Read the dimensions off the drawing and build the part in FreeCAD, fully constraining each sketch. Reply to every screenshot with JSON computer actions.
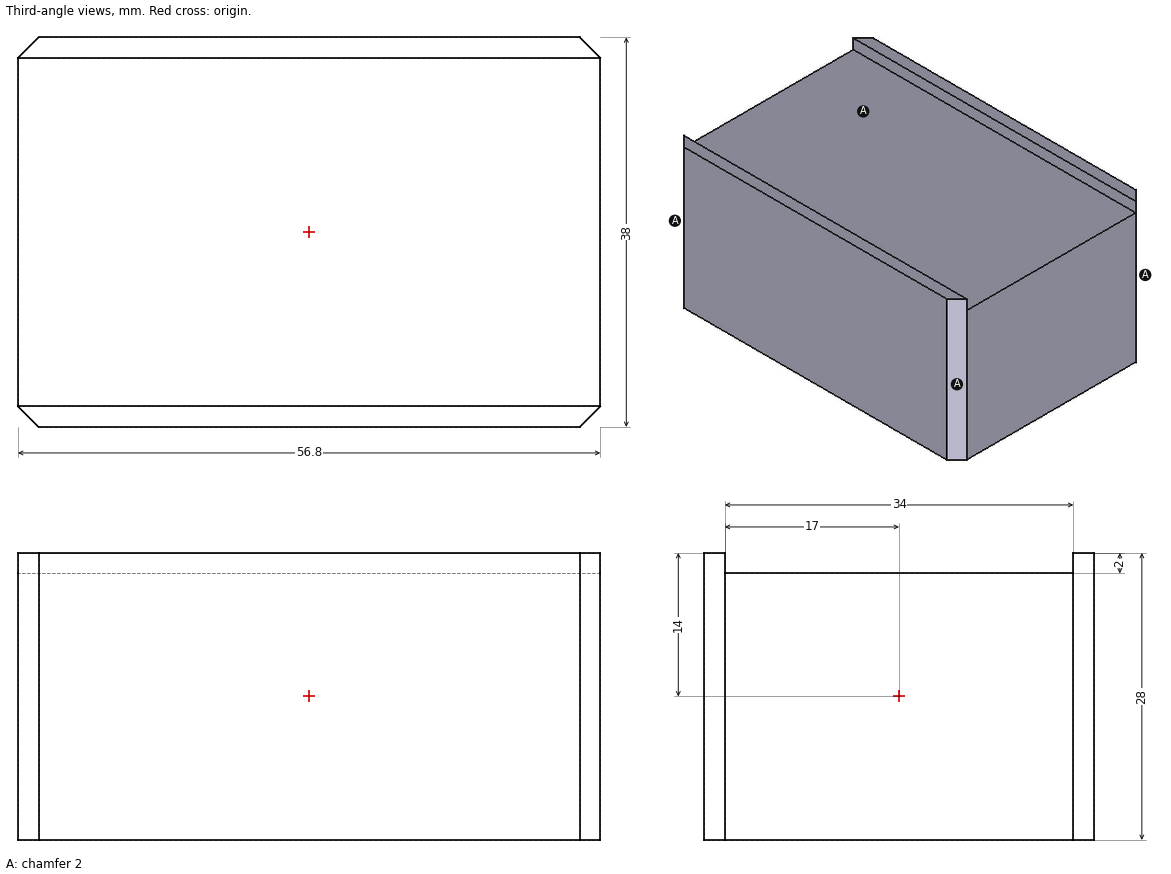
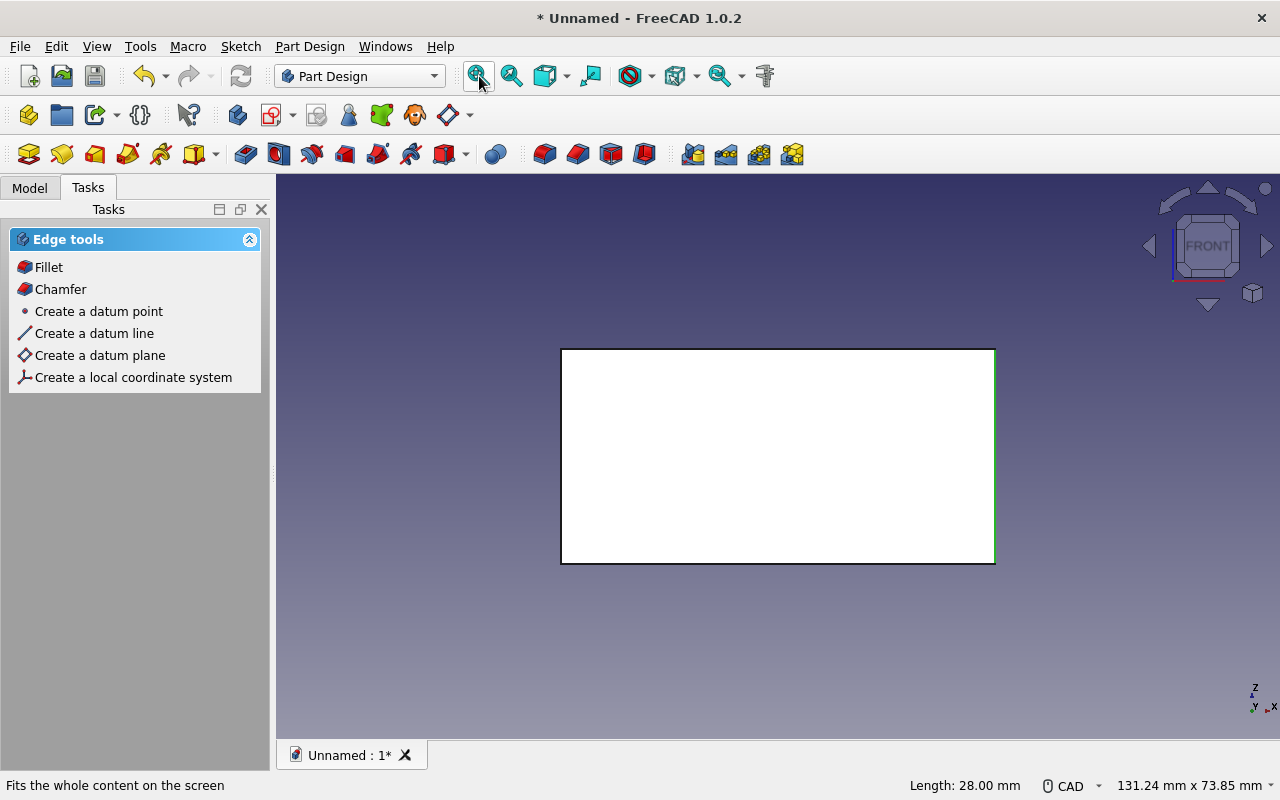
{"action": "left_click", "coordinate": [561, 456], "text": "ctrl"}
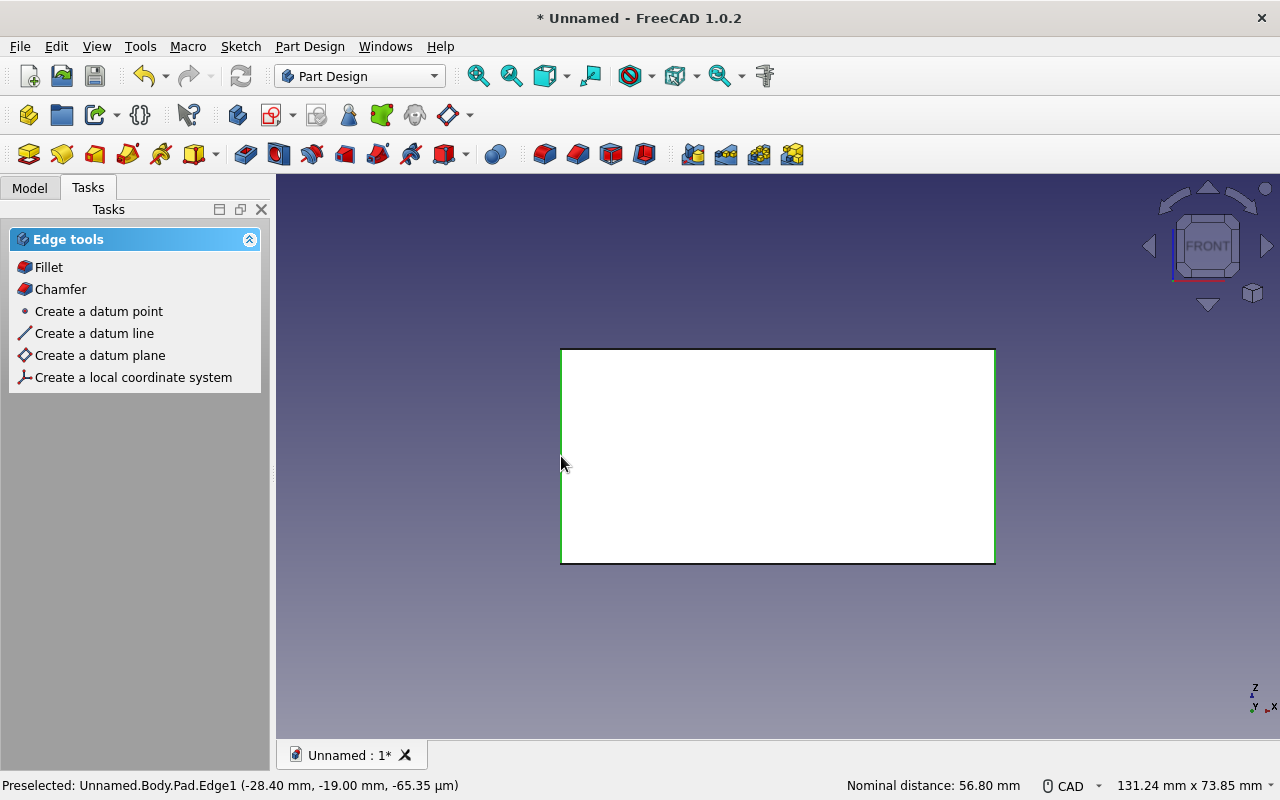
{"action": "key", "text": "3"}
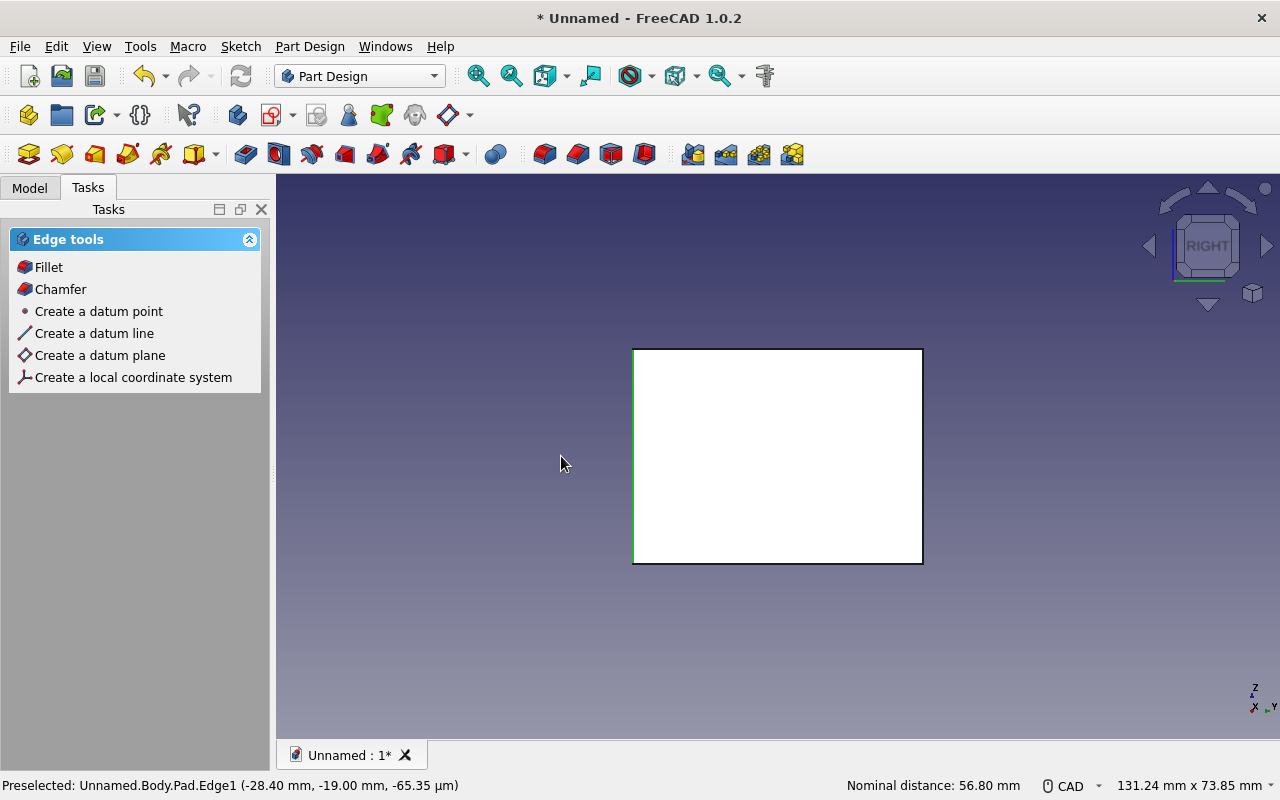
{"action": "left_click", "coordinate": [479, 76]}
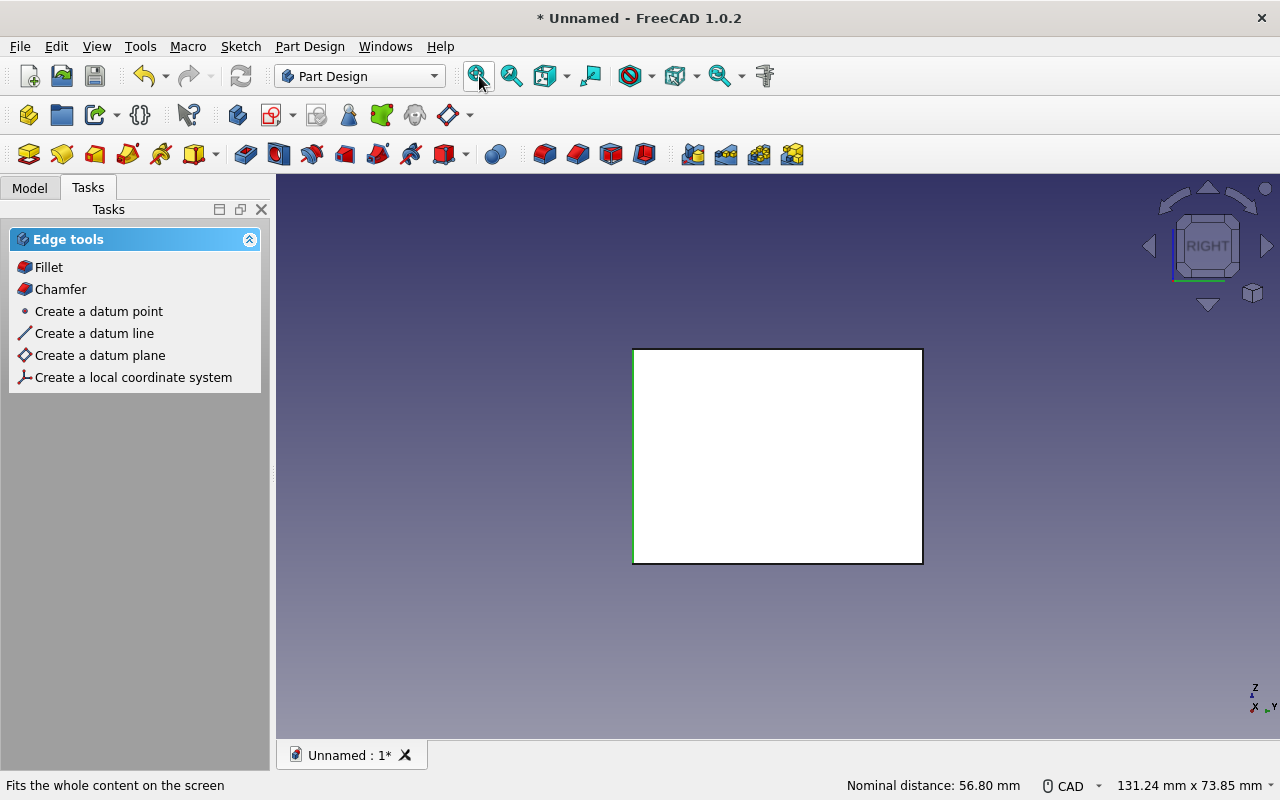
{"action": "left_click", "coordinate": [923, 455], "text": "ctrl"}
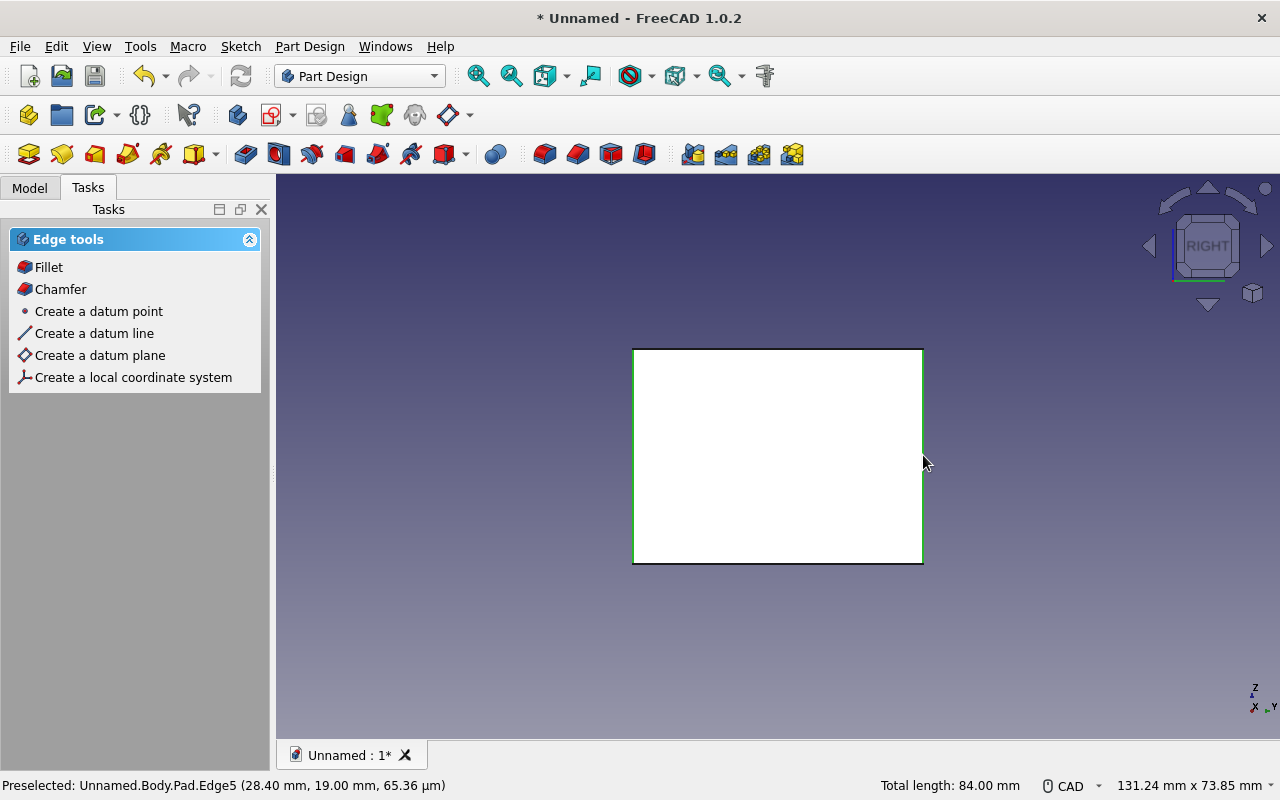
{"action": "key", "text": "5"}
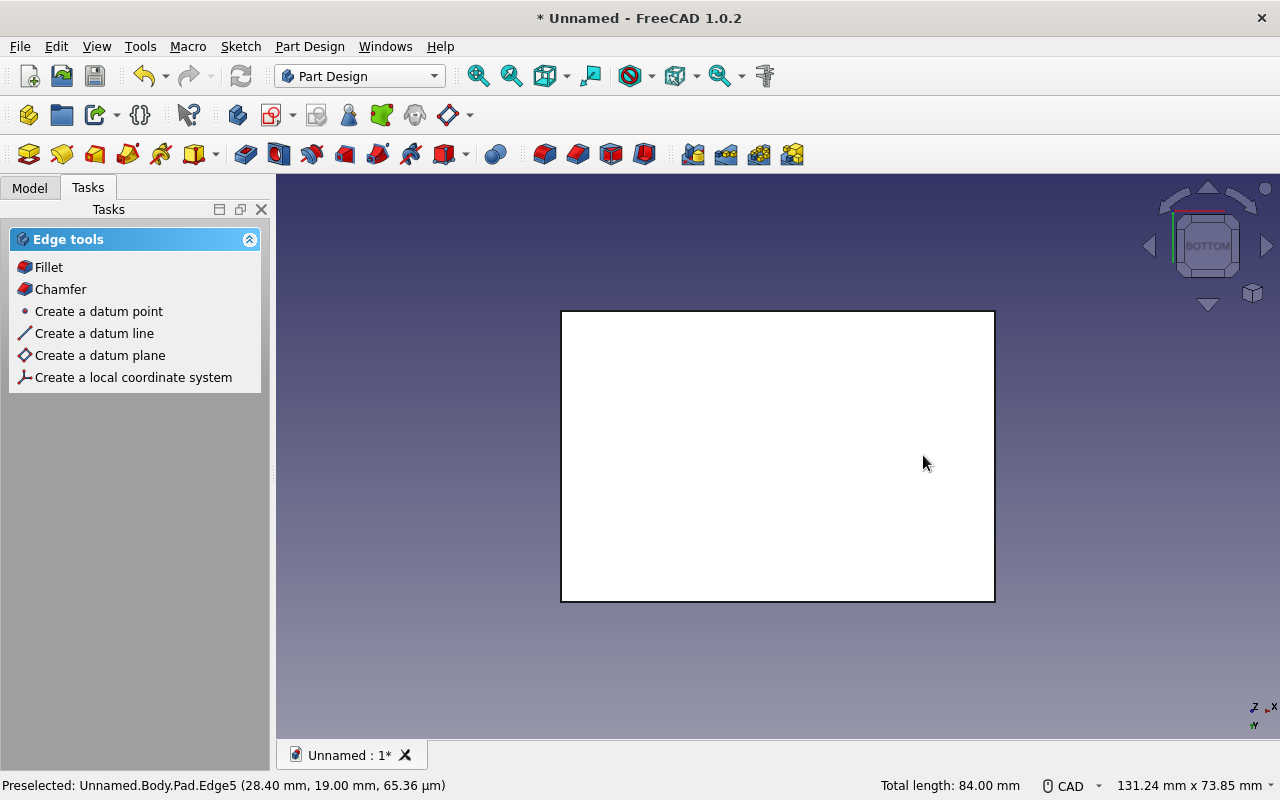
{"action": "key", "text": "4"}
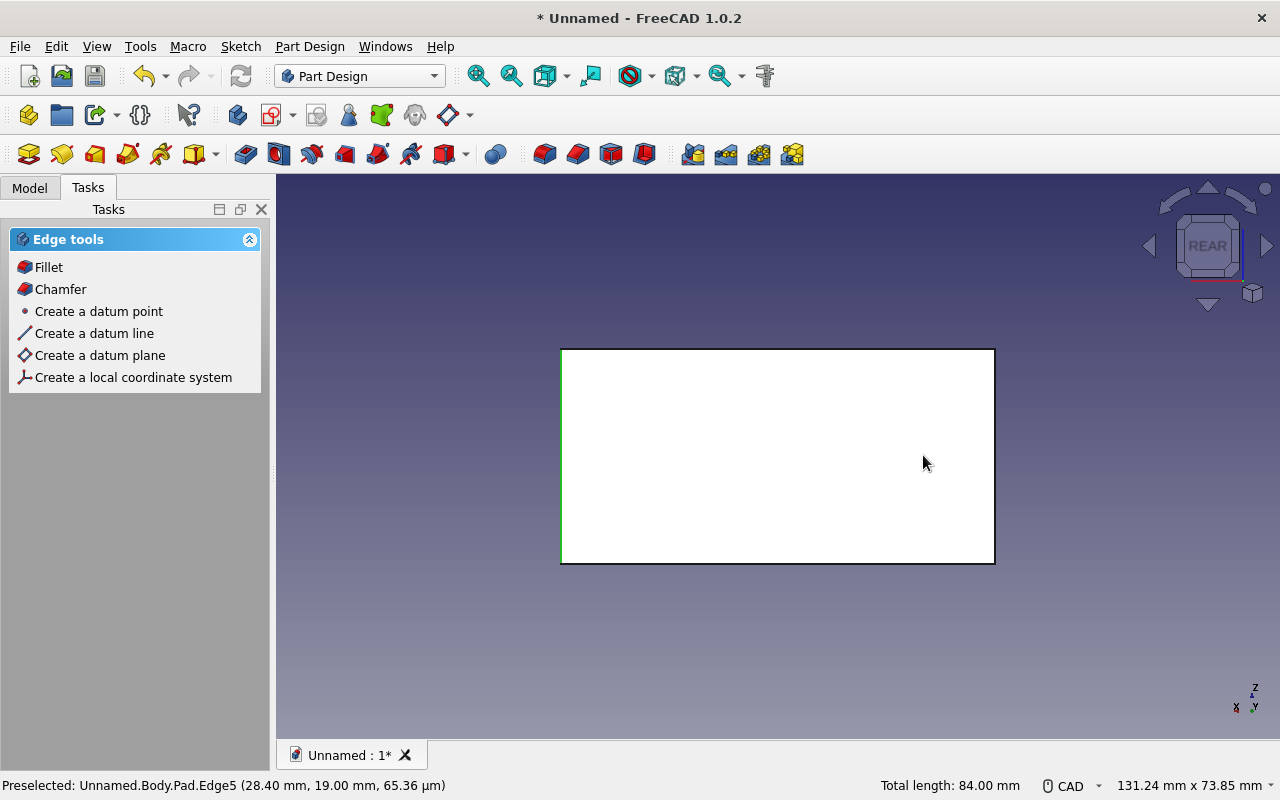
{"action": "left_click", "coordinate": [479, 76]}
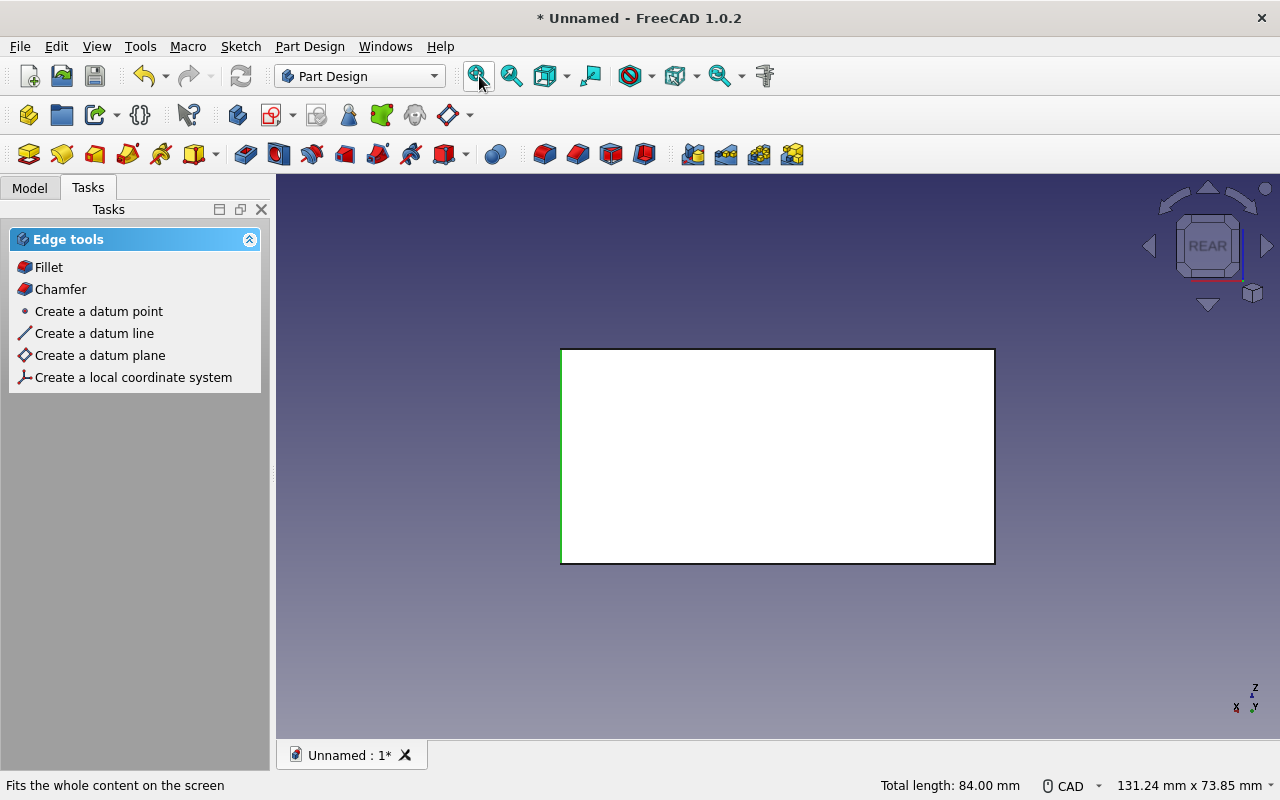
{"action": "left_click", "coordinate": [995, 456], "text": "ctrl"}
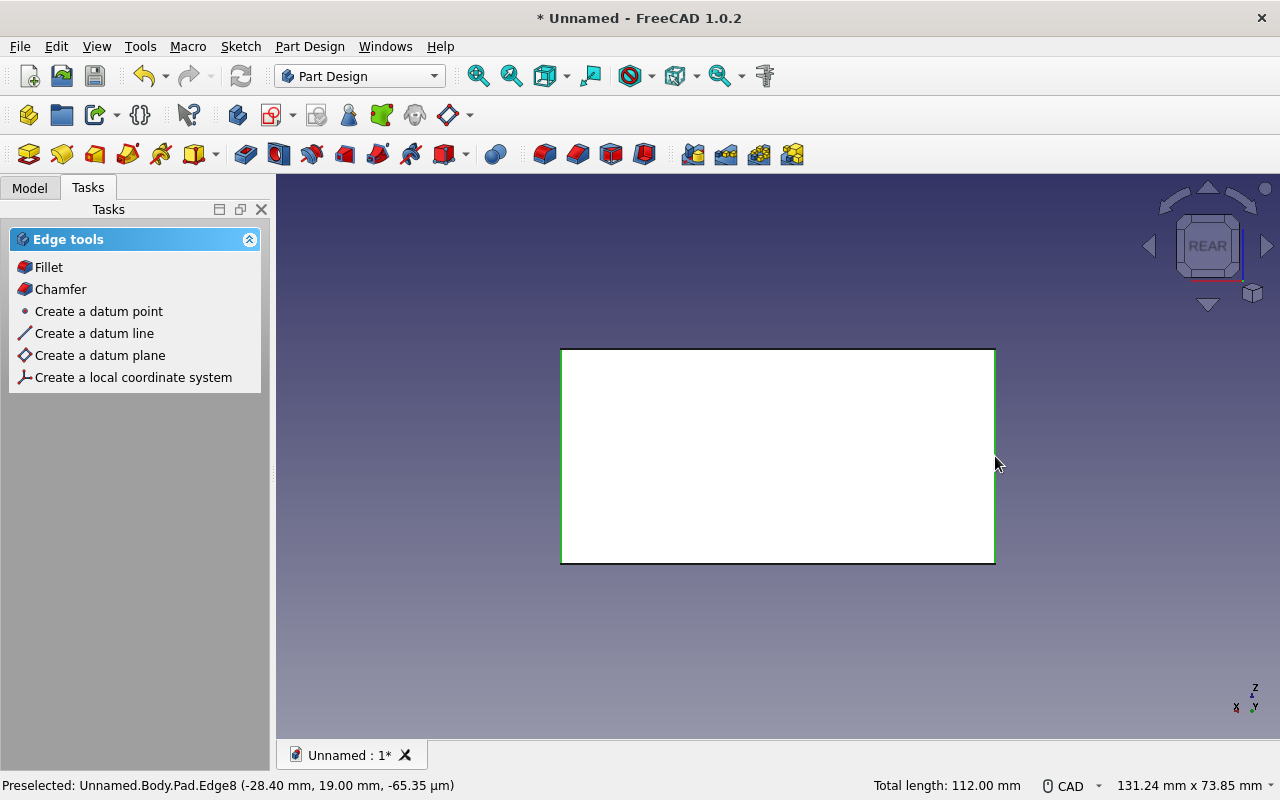
{"action": "left_click", "coordinate": [578, 154]}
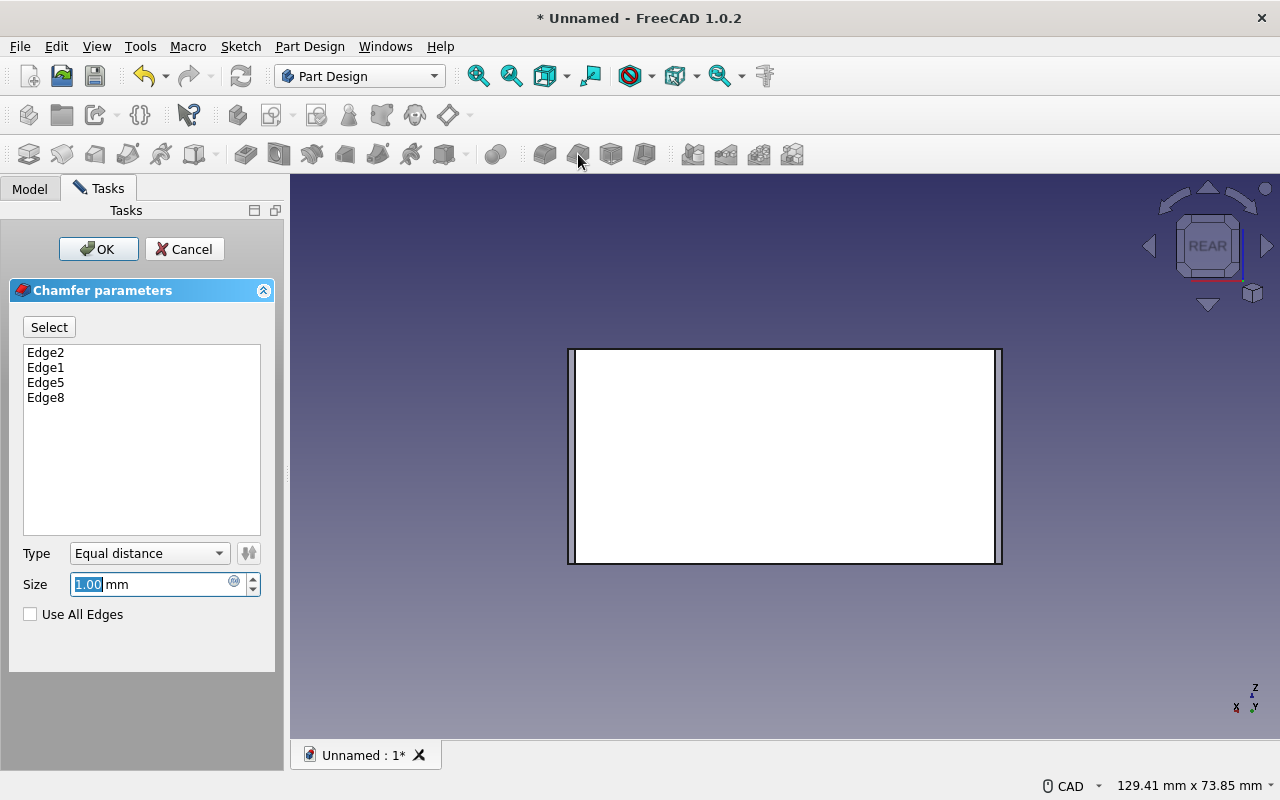
{"action": "type", "text": "2"}
{"action": "key", "text": "Tab"}